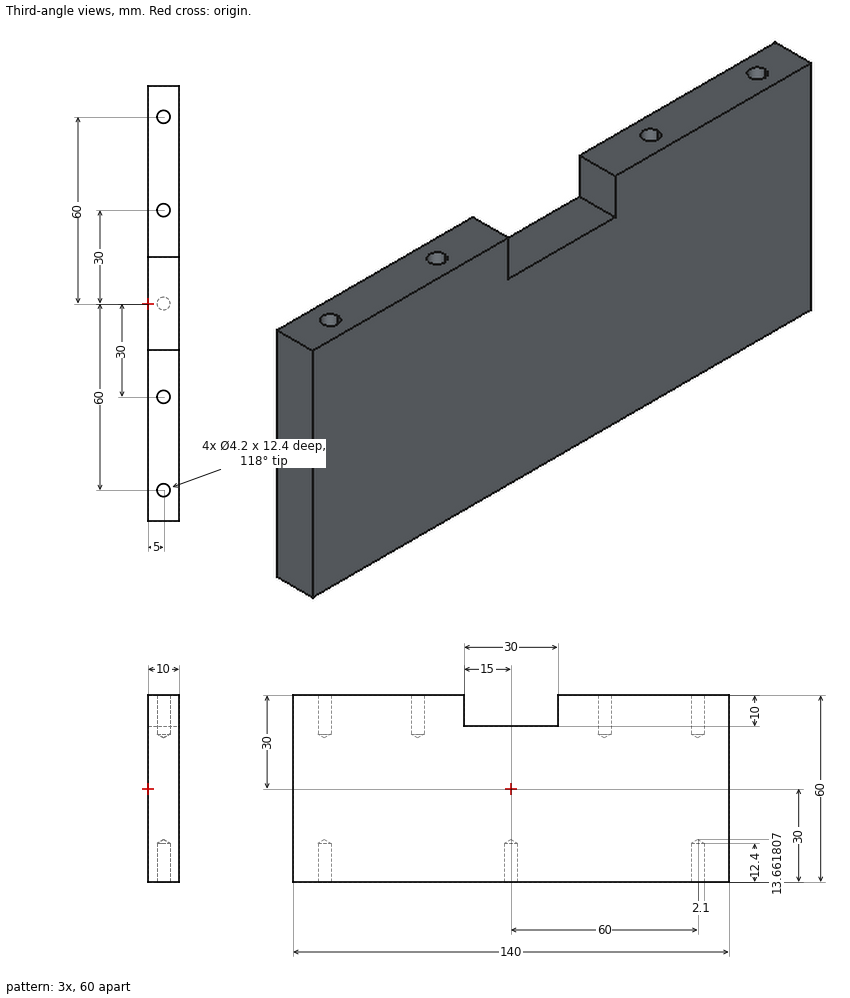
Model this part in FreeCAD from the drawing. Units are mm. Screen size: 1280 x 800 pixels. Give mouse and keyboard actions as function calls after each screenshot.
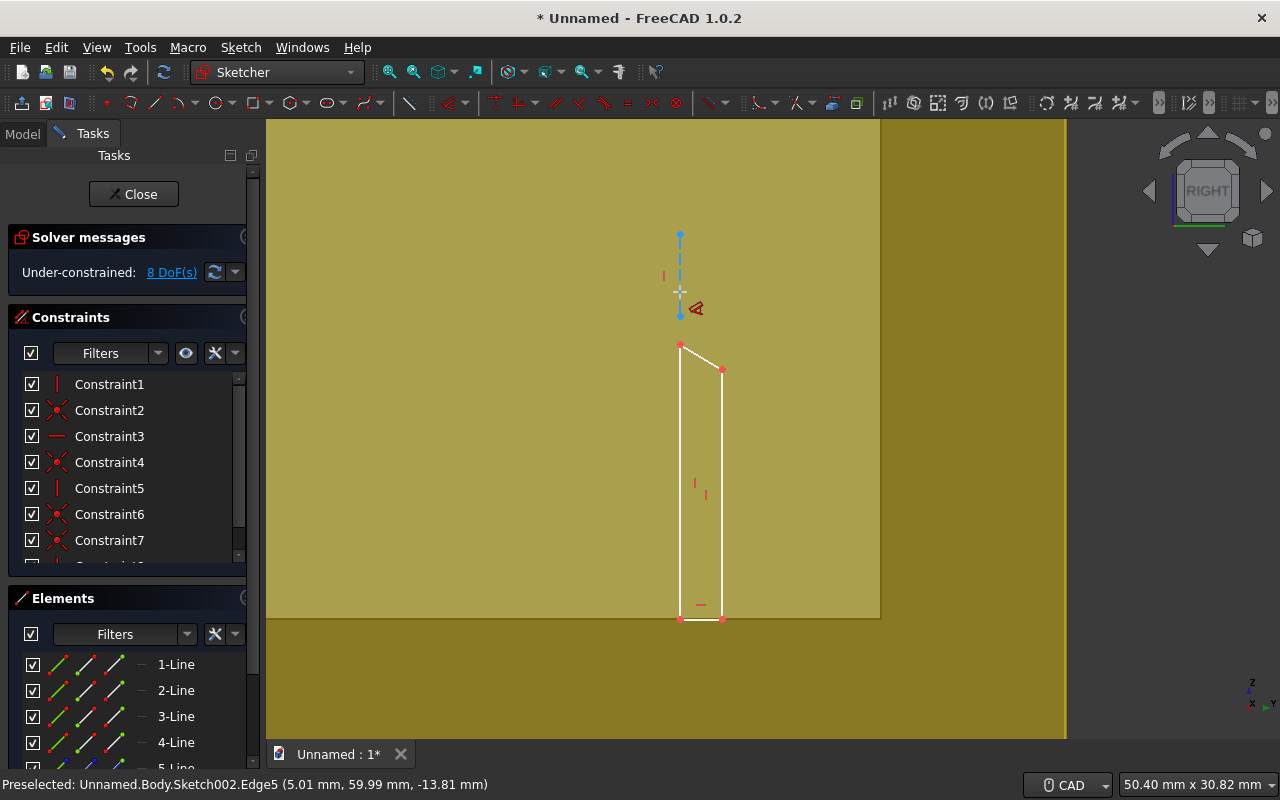
click(693, 620)
click(701, 654)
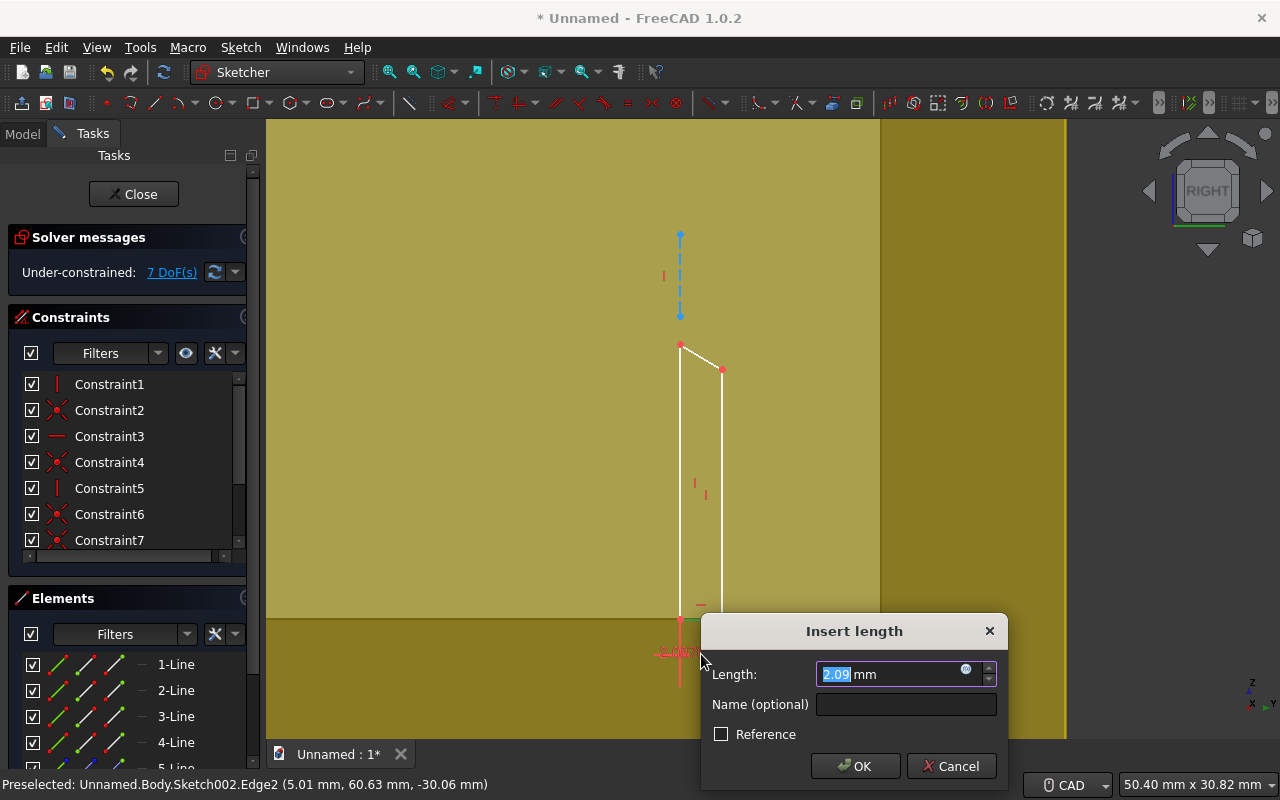
text(2.1)
key(Return)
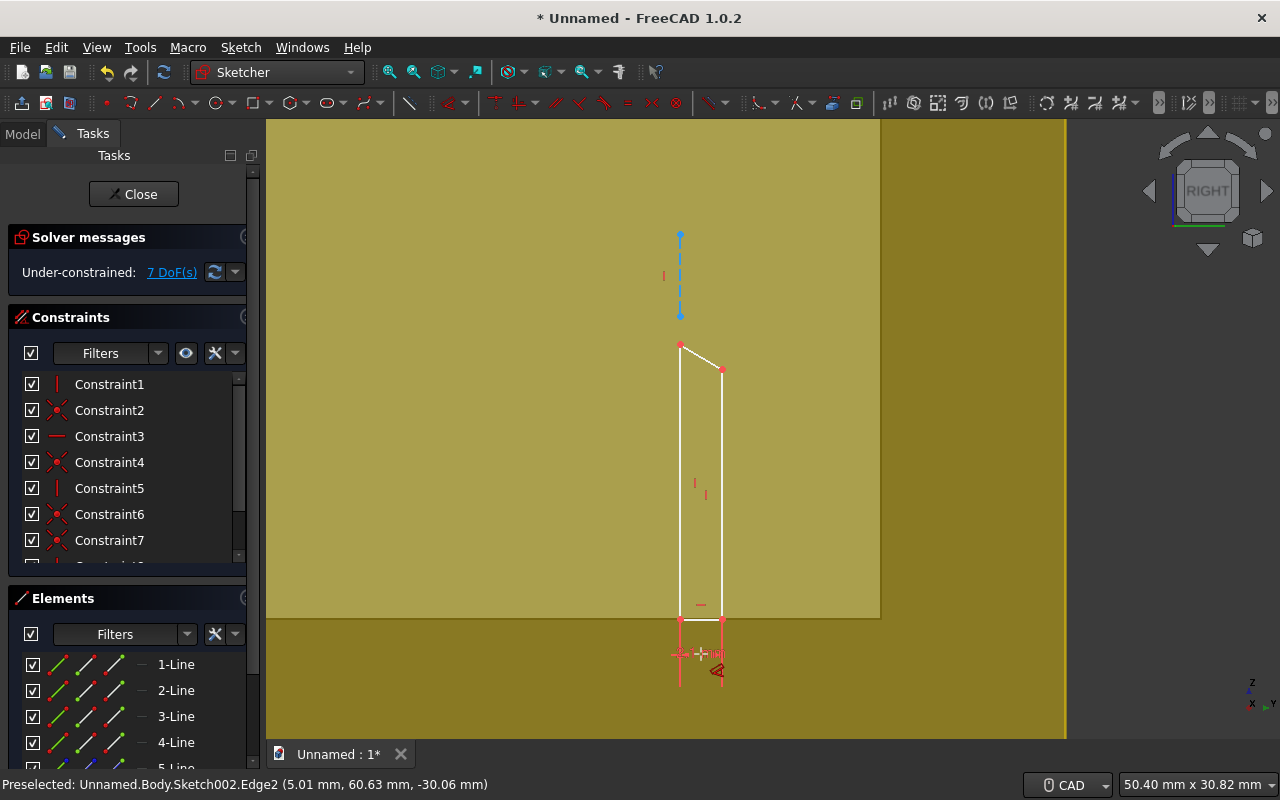
click(680, 345)
click(487, 379)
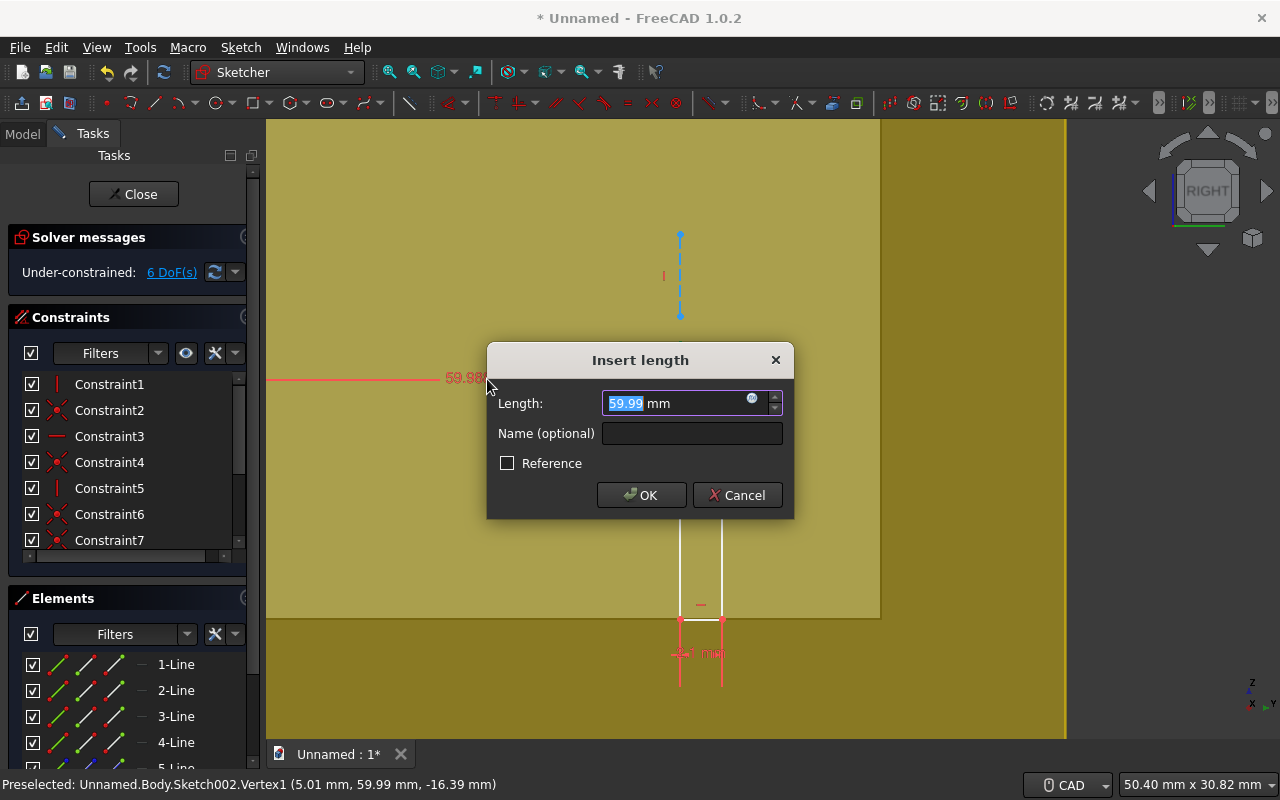
text(60)
key(Return)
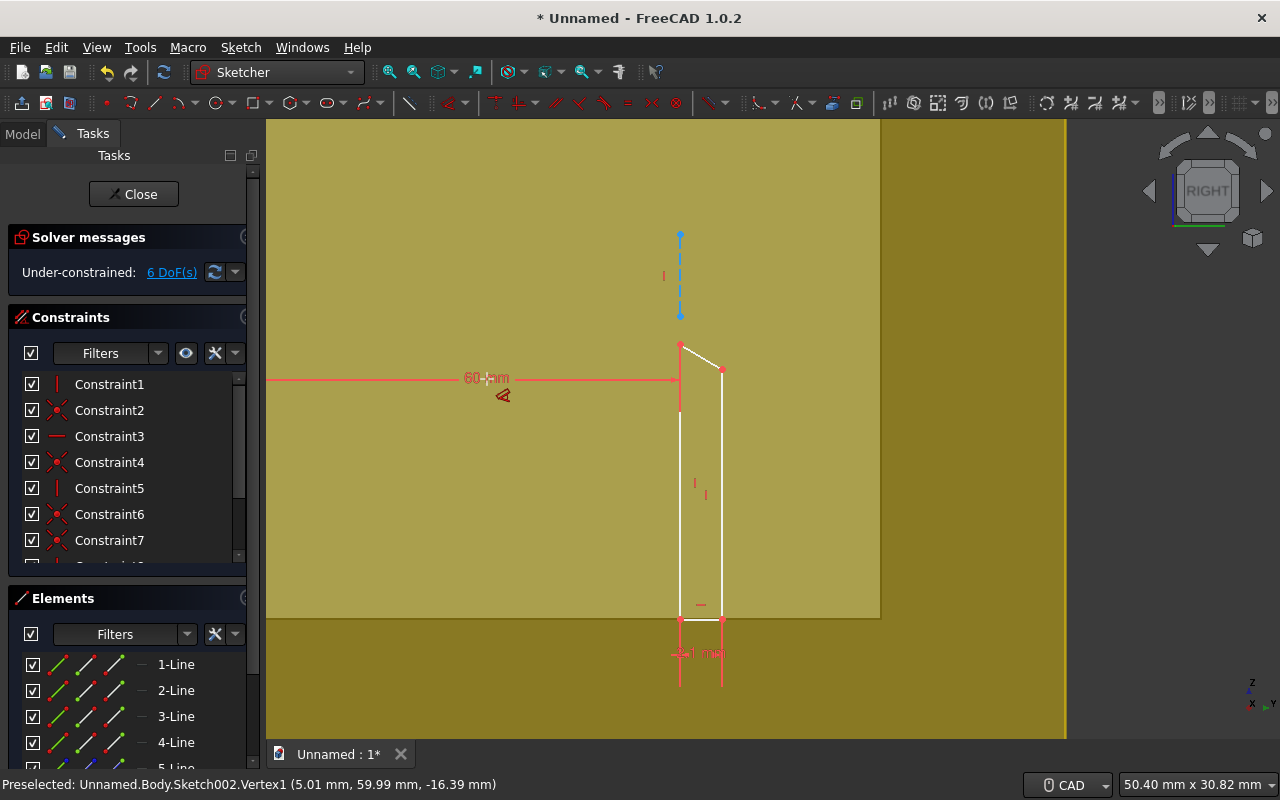
click(680, 620)
click(714, 275)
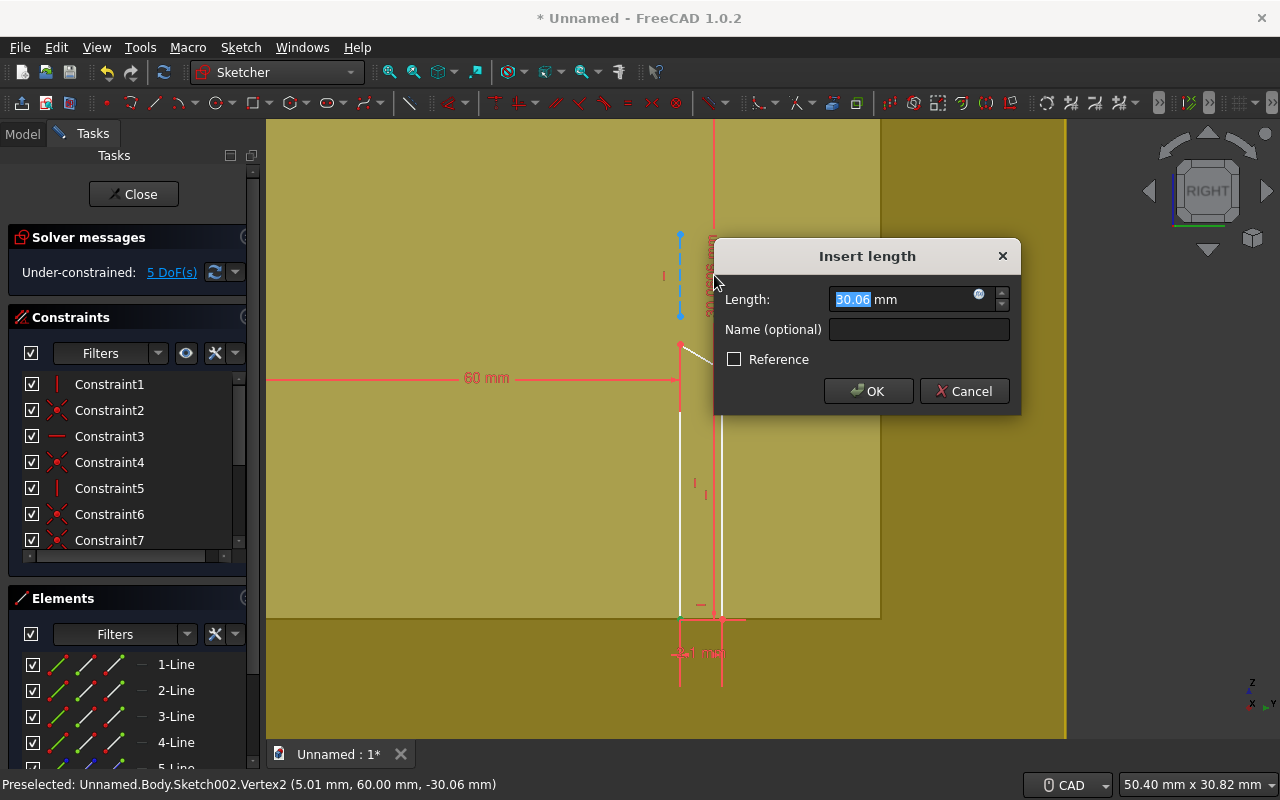
text(30)
key(Return)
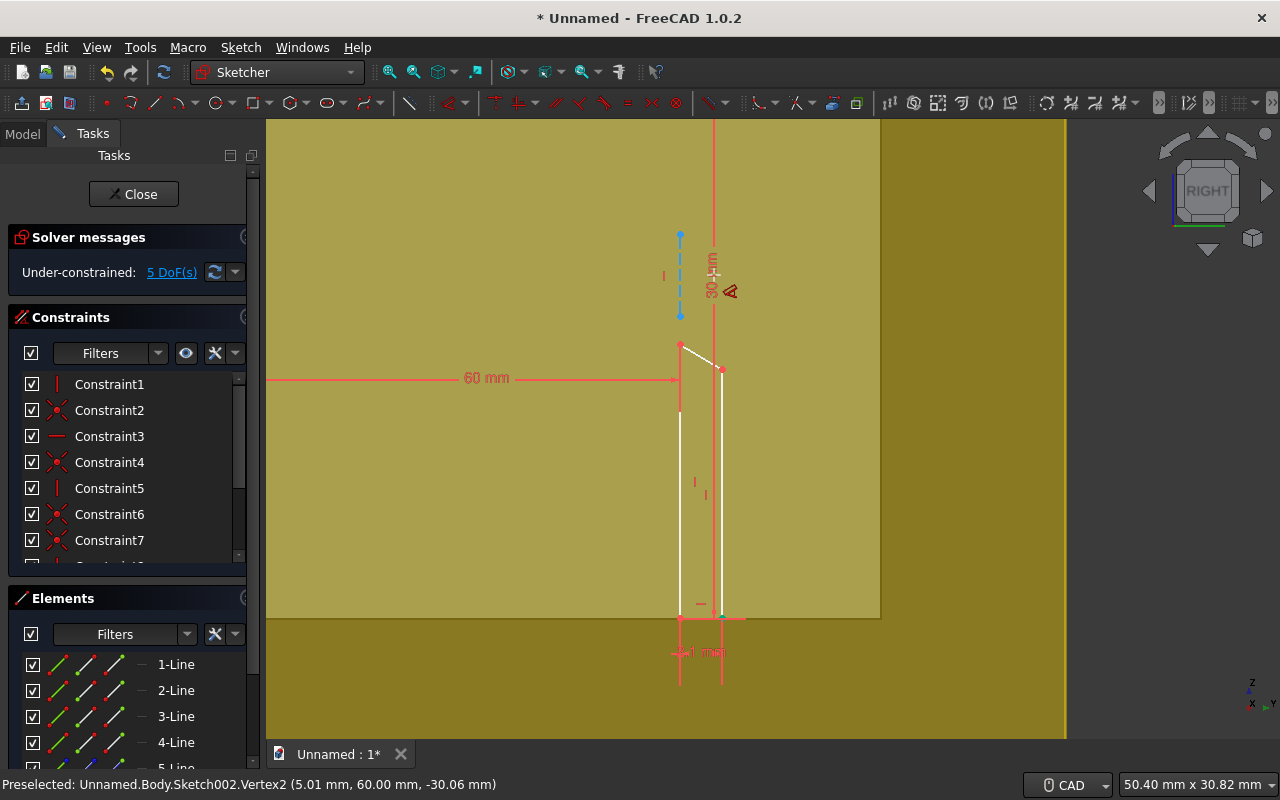
click(680, 317)
click(487, 351)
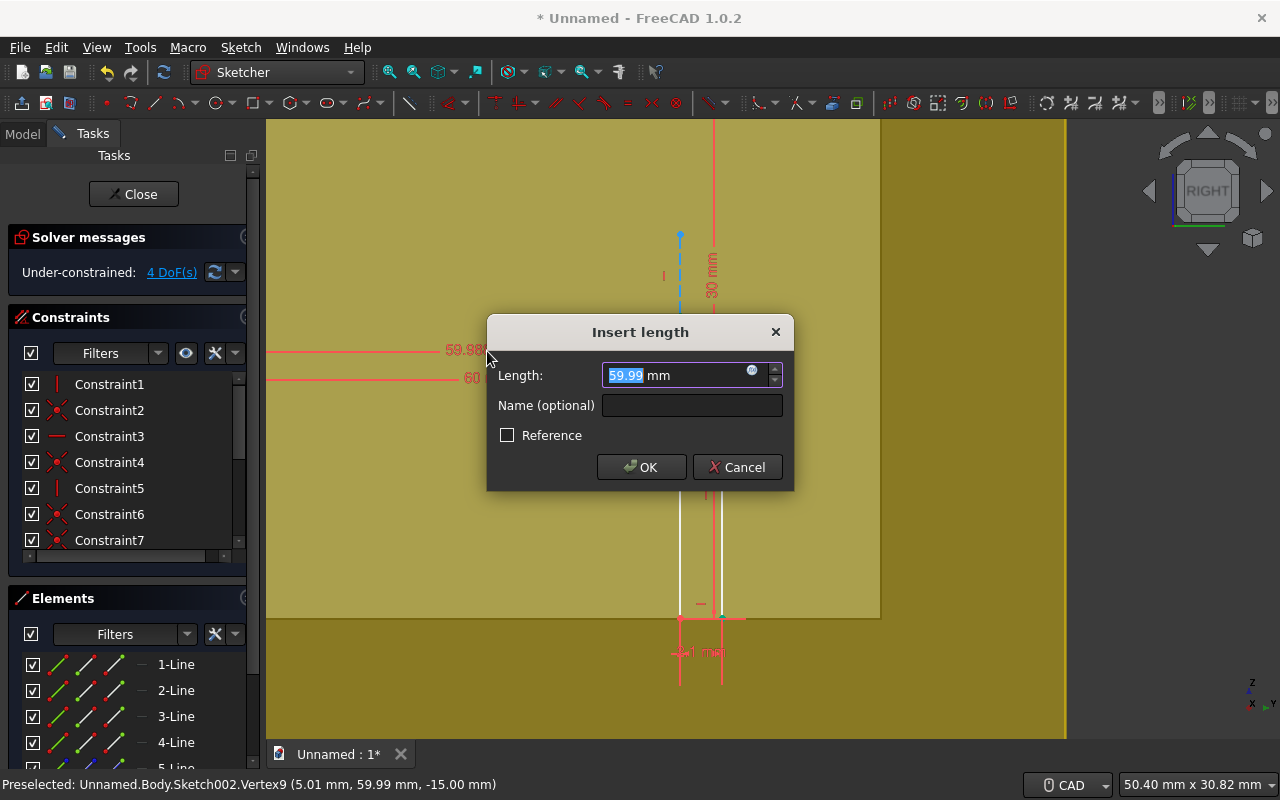
text(60)
key(Return)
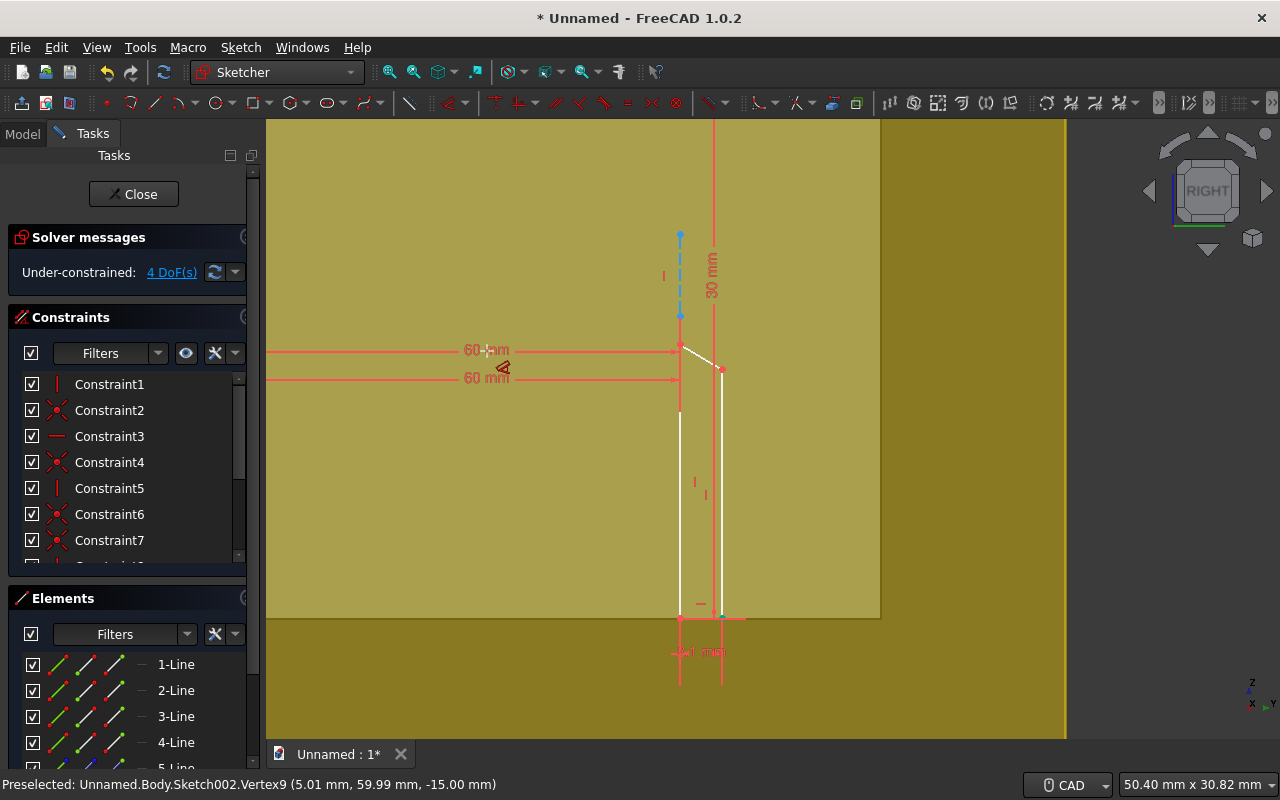
click(722, 544)
click(756, 494)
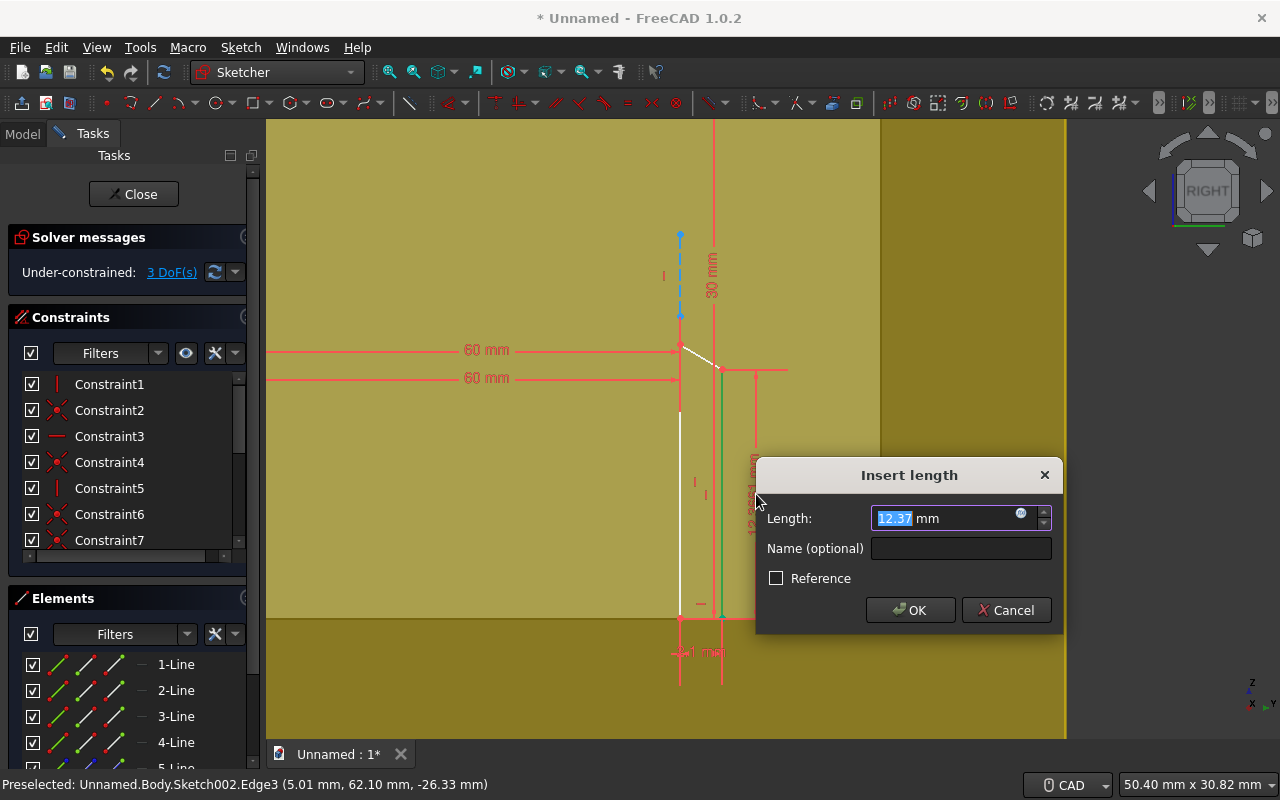
text(12.4)
key(Return)